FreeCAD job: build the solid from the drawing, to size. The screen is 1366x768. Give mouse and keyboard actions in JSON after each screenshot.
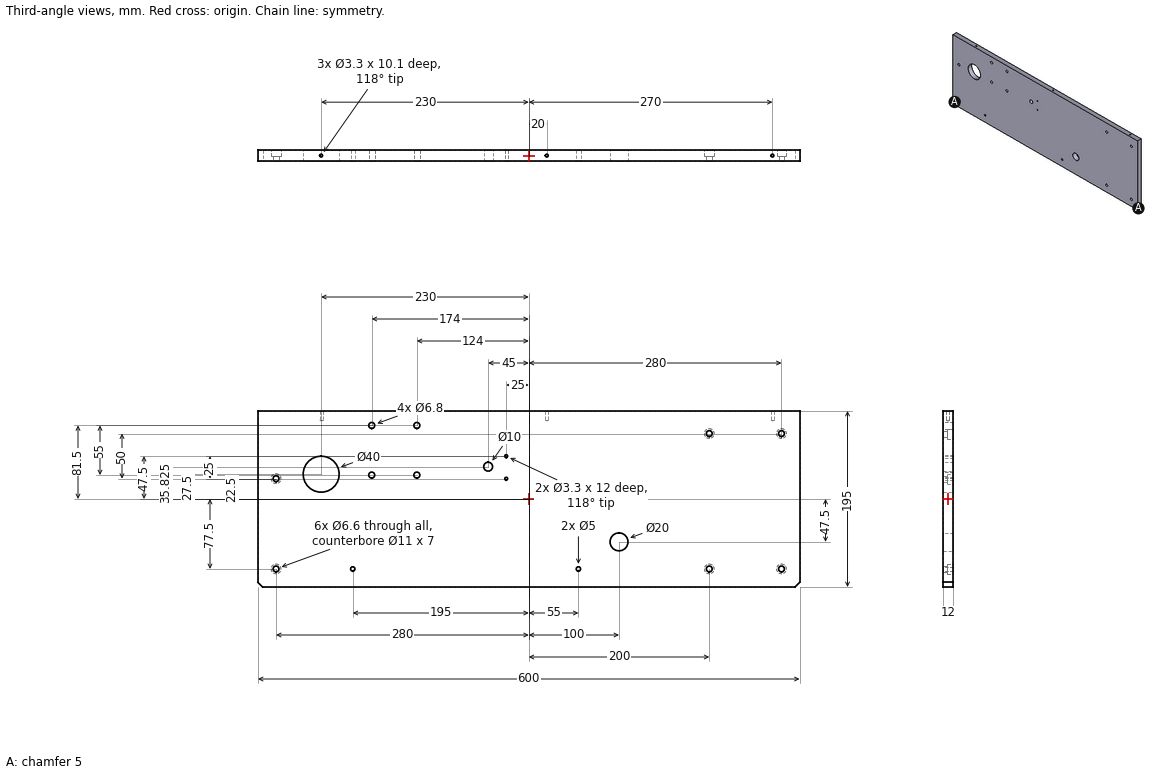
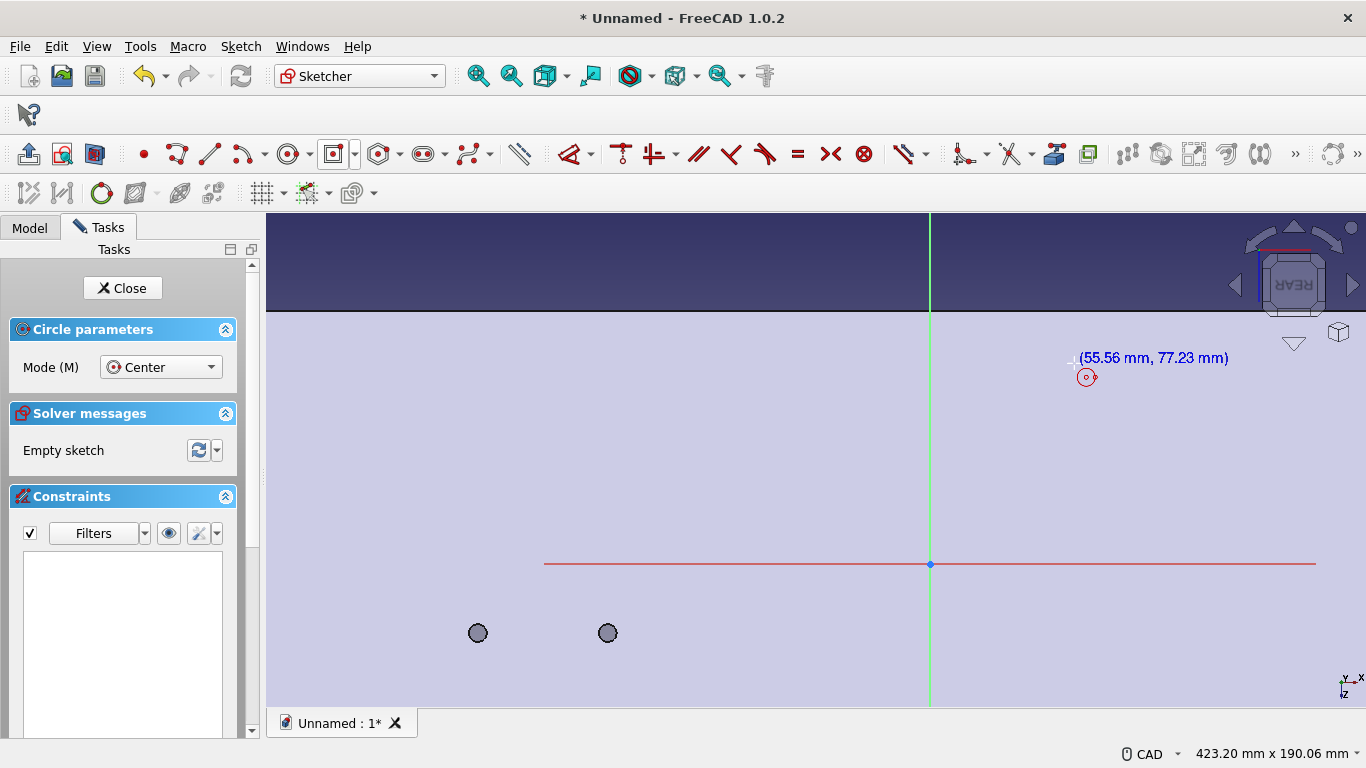
{"action": "left_click", "coordinate": [1073, 363]}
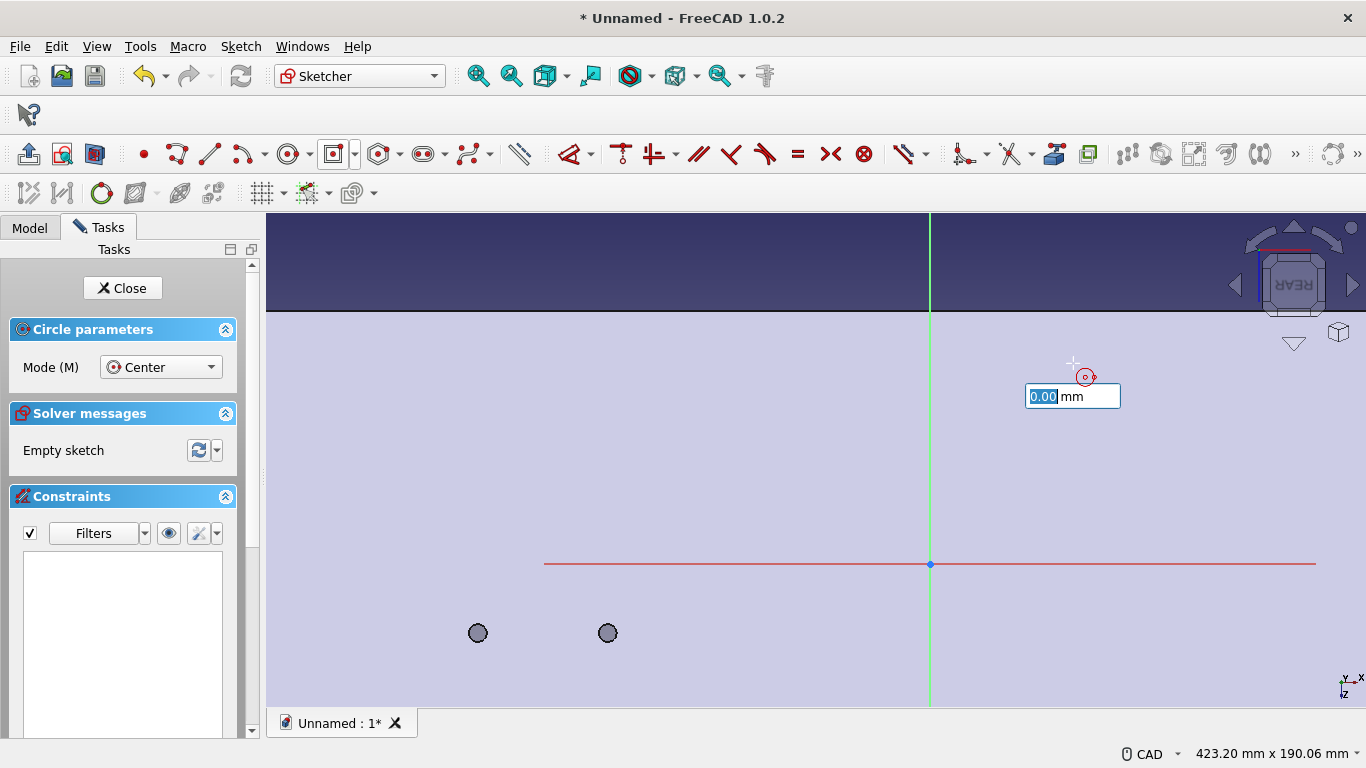
{"action": "scroll", "coordinate": [1078, 358], "scroll_direction": "up", "scroll_amount": 5}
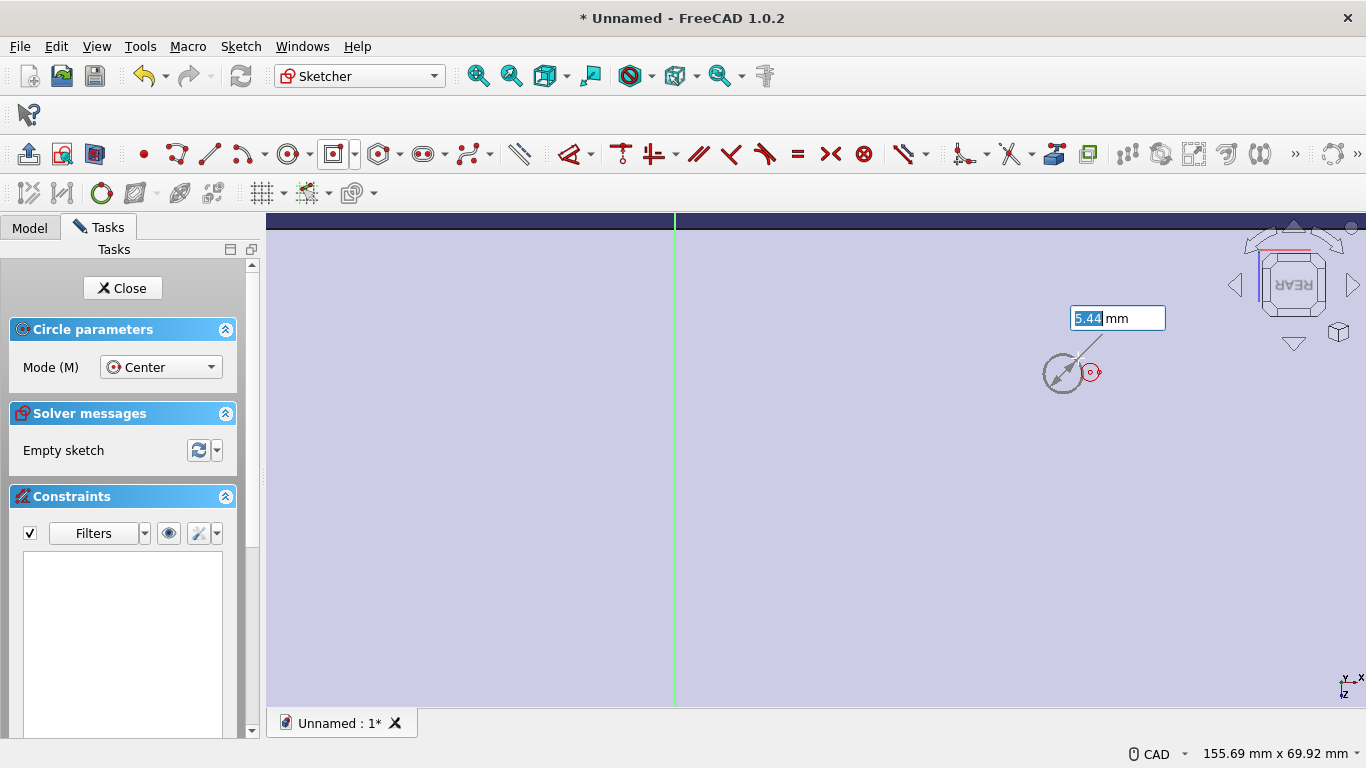
{"action": "left_click", "coordinate": [1076, 358]}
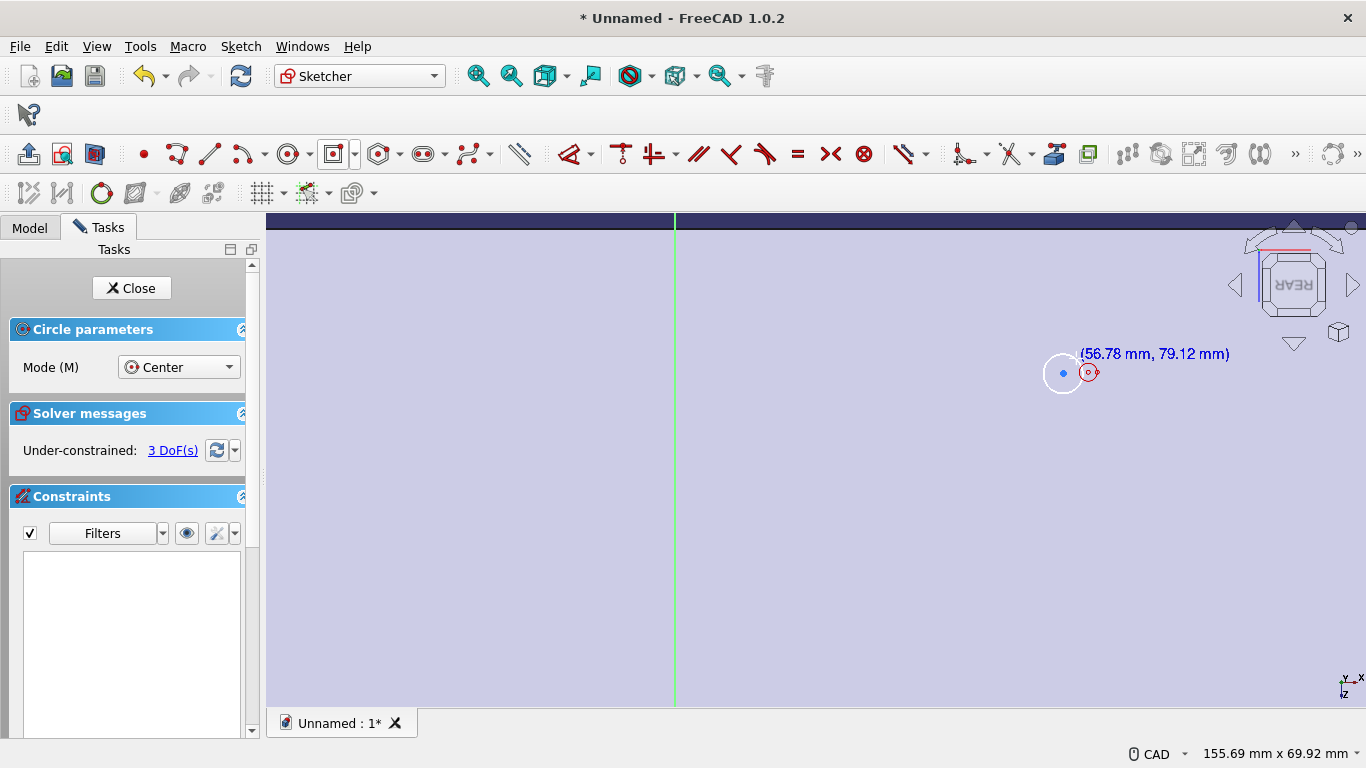
{"action": "scroll", "coordinate": [1078, 358], "scroll_direction": "down", "scroll_amount": 5}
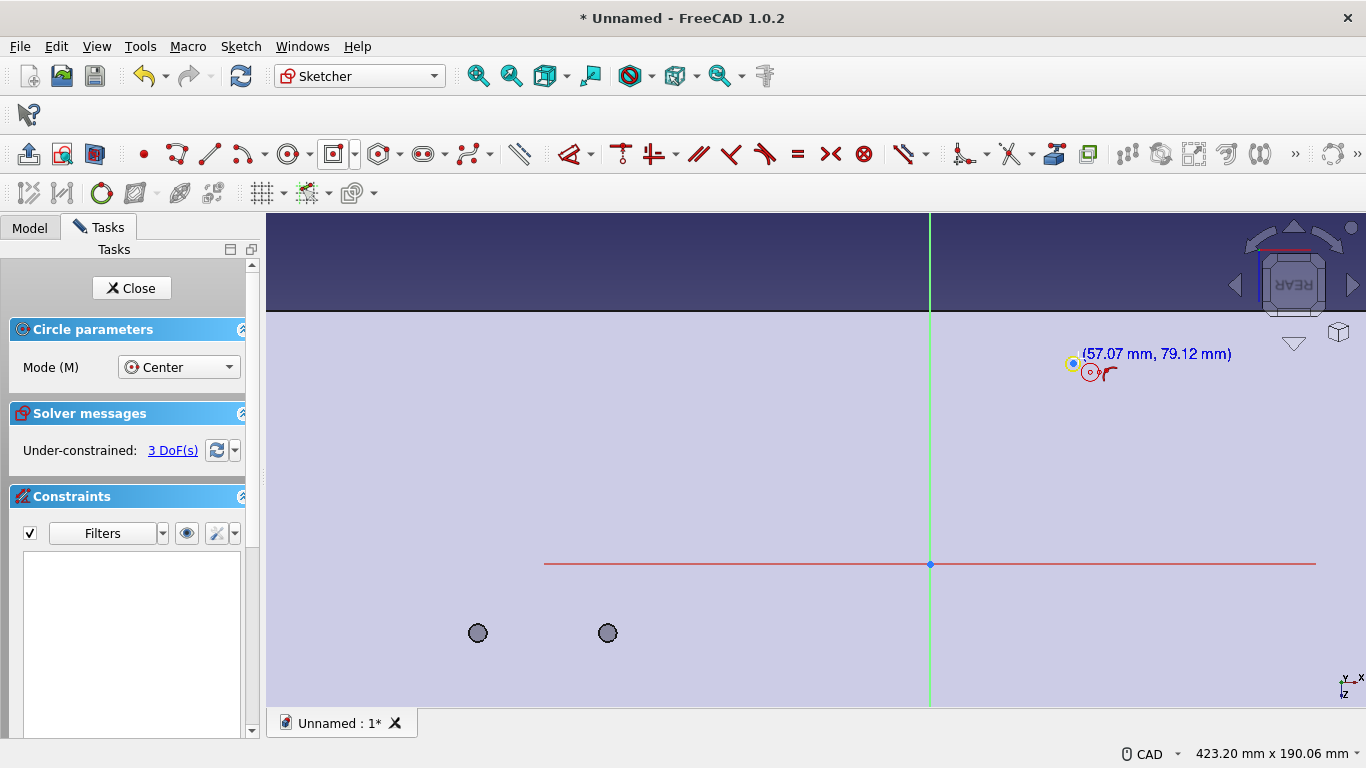
{"action": "scroll", "coordinate": [423, 363], "scroll_direction": "up", "scroll_amount": 7}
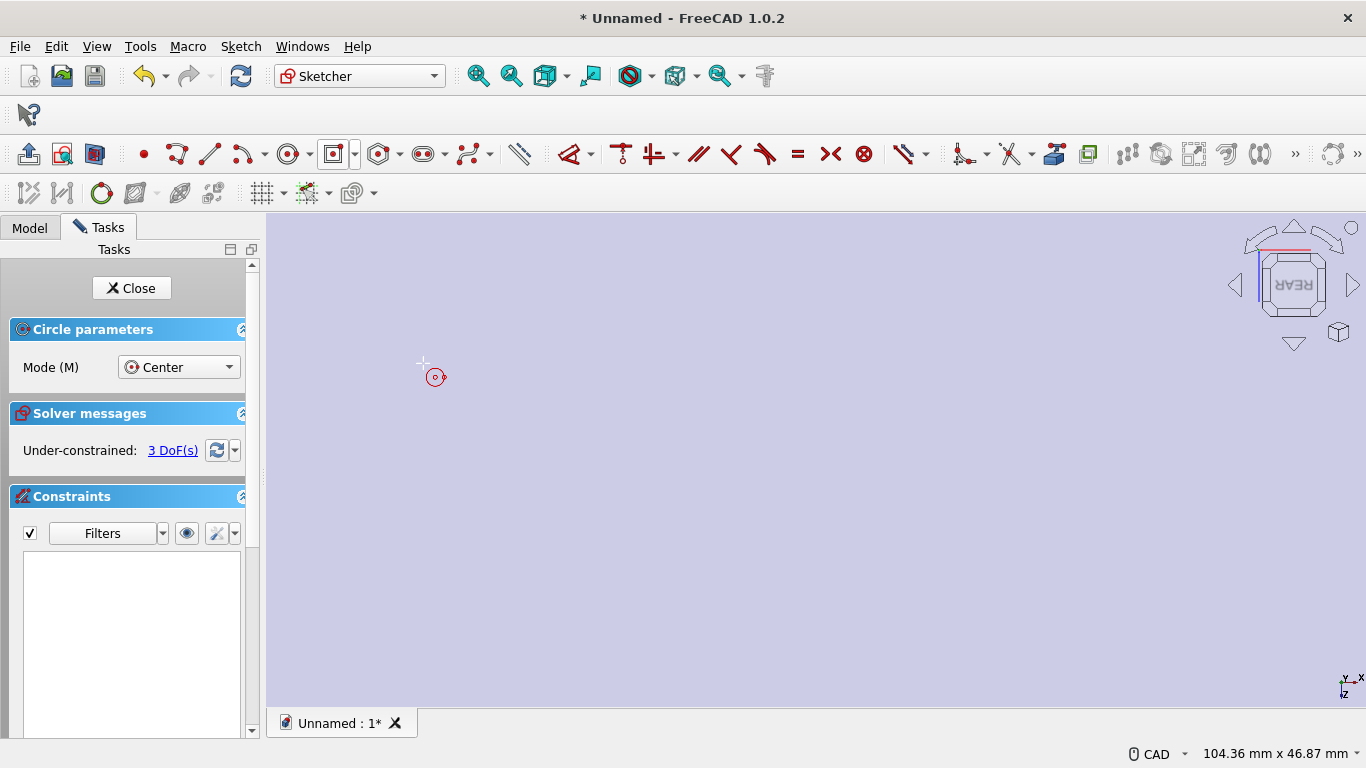
{"action": "scroll", "coordinate": [422, 363], "scroll_direction": "down", "scroll_amount": 7}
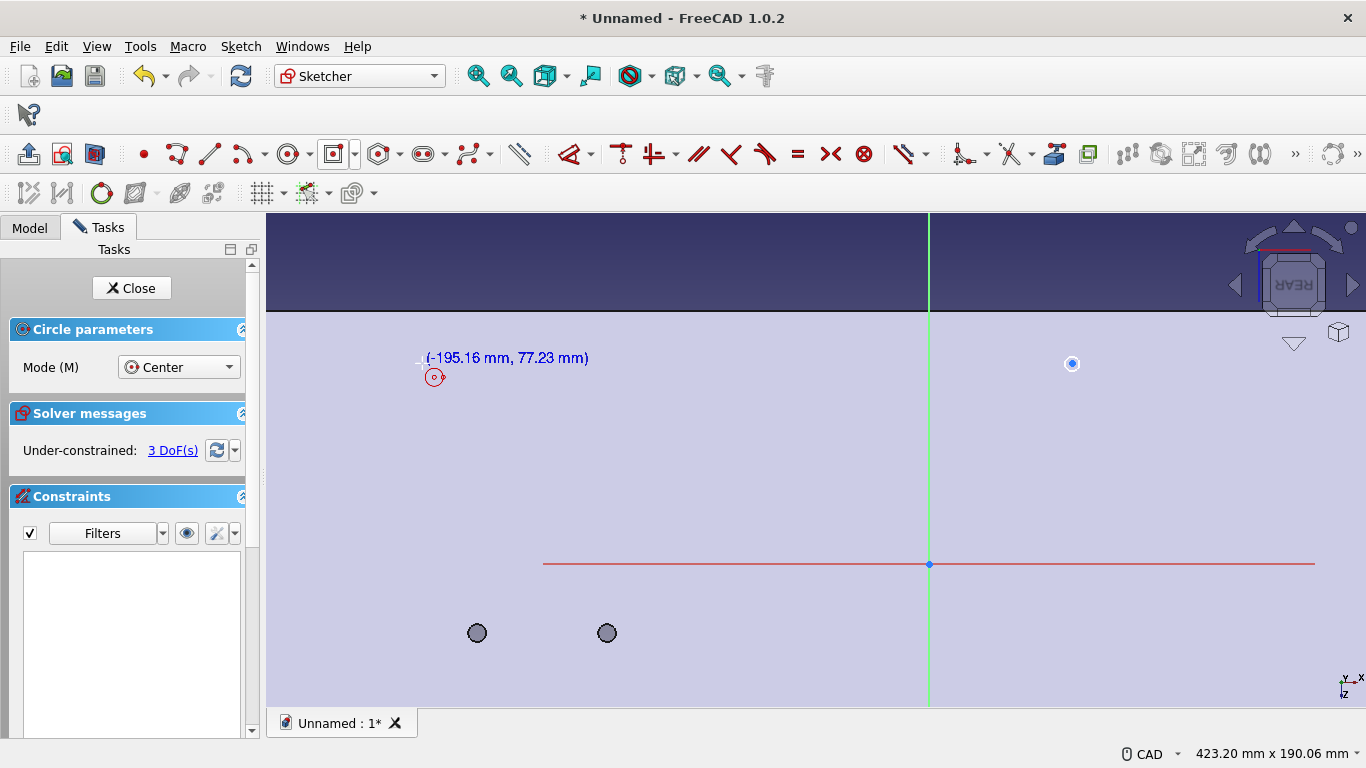
{"action": "left_click", "coordinate": [423, 363]}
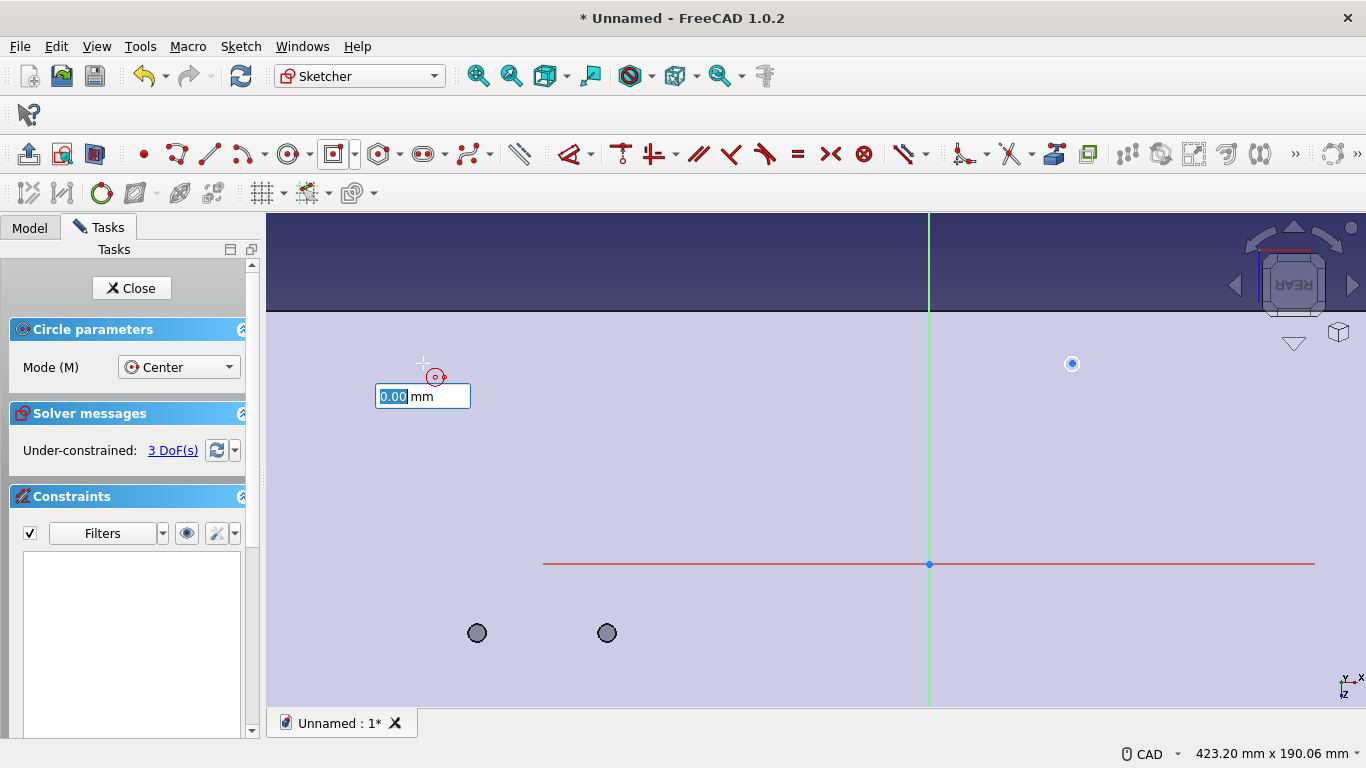
{"action": "scroll", "coordinate": [427, 358], "scroll_direction": "up", "scroll_amount": 5}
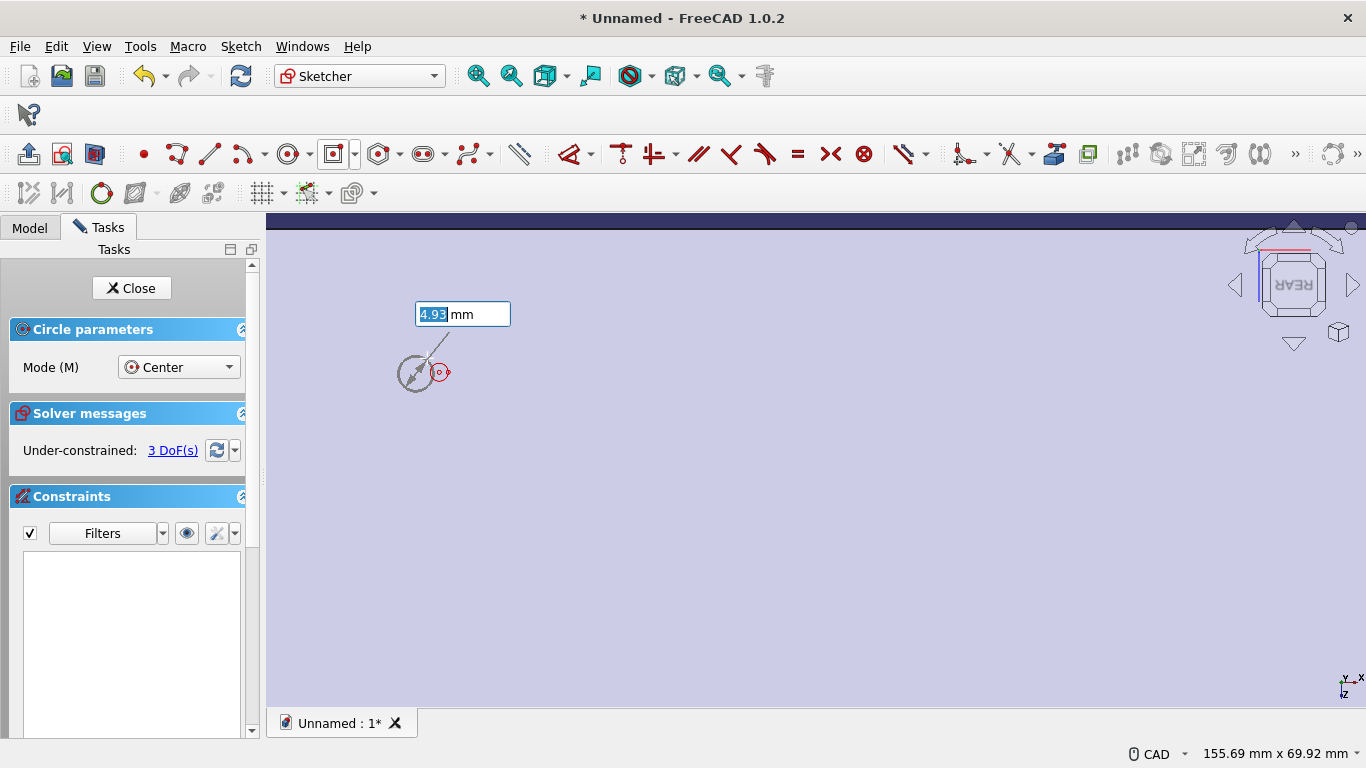
{"action": "left_click", "coordinate": [427, 358]}
{"action": "key", "text": "Escape"}